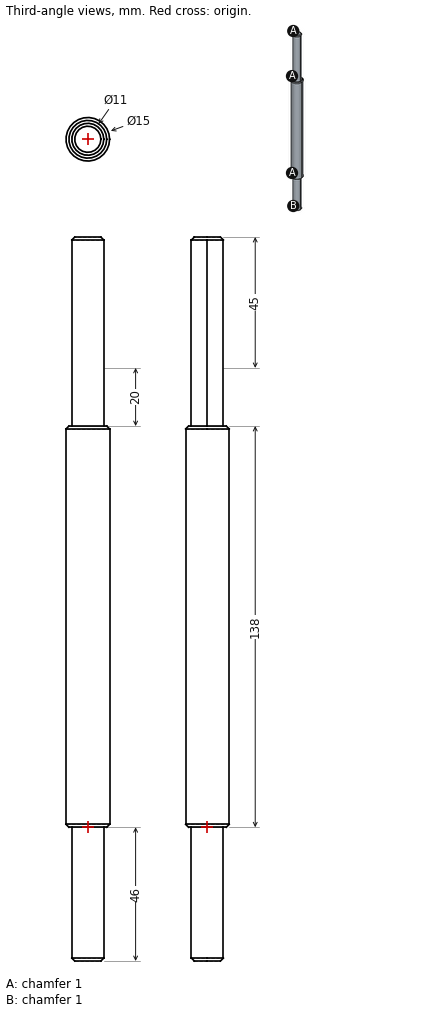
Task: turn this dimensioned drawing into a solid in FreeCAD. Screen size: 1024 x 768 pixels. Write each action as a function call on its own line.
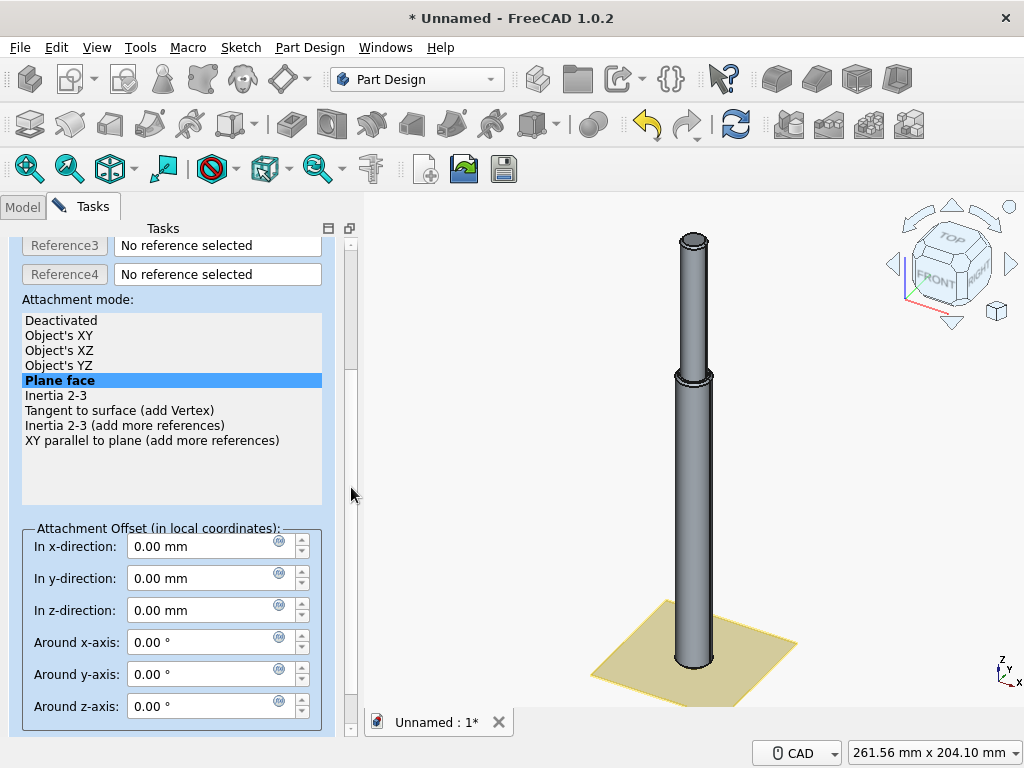
triple_click(210, 610)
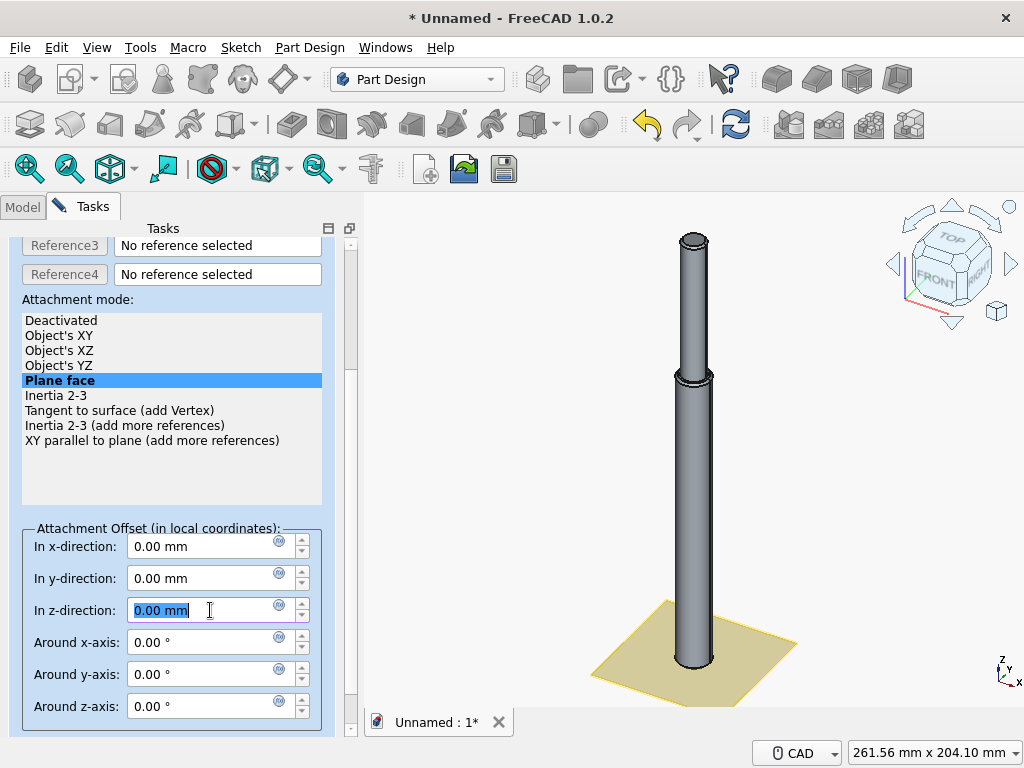
text(-46)
key(Tab)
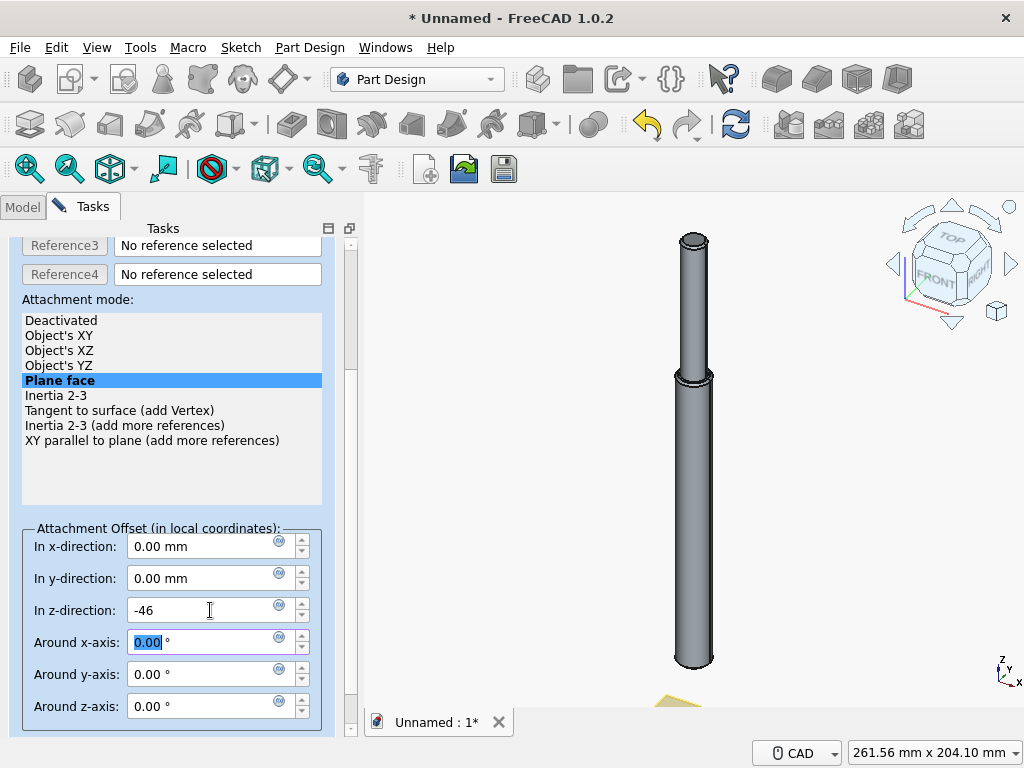
scroll(351, 487, up, 4)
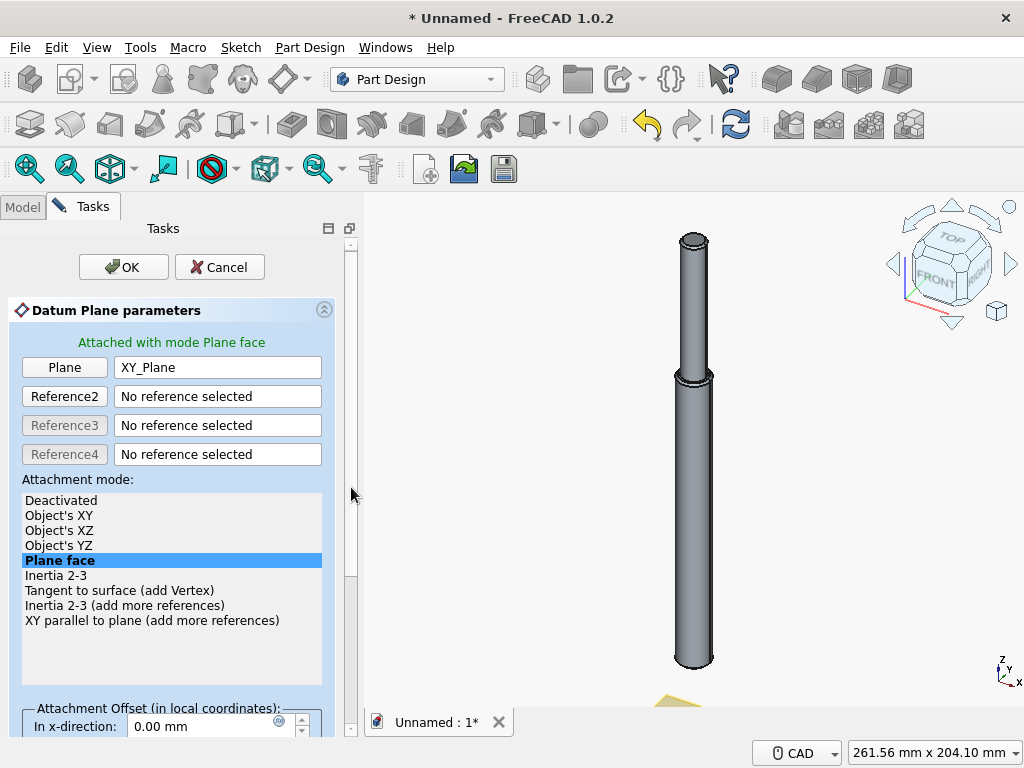
click(124, 267)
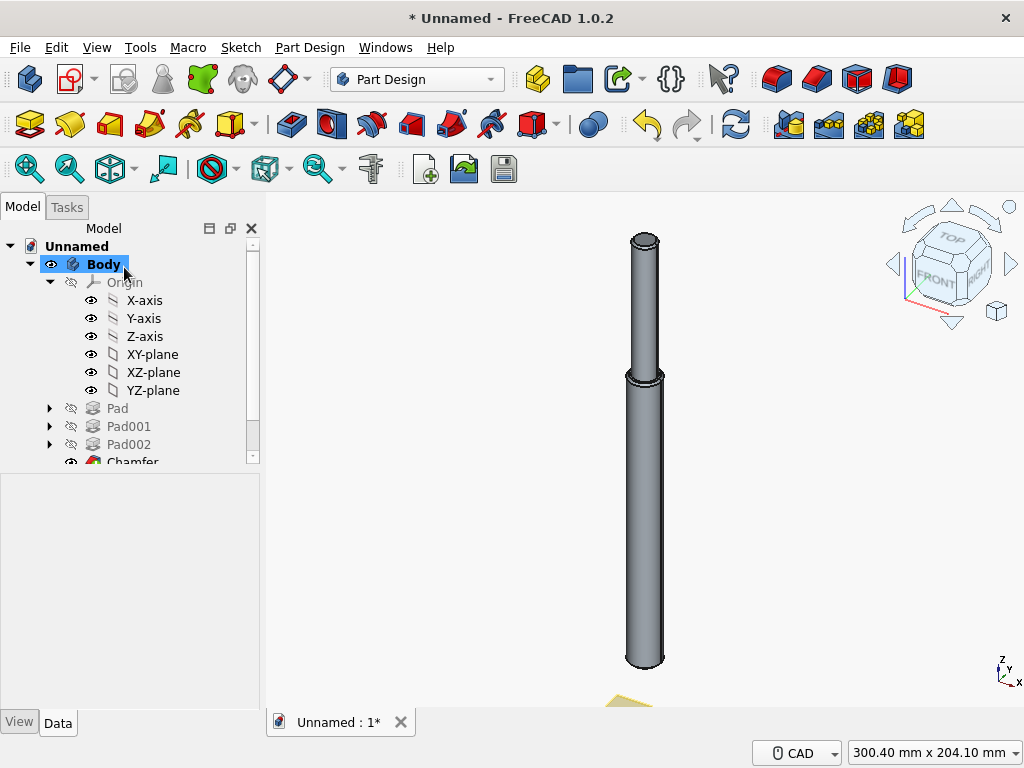
scroll(100, 350, down, 3)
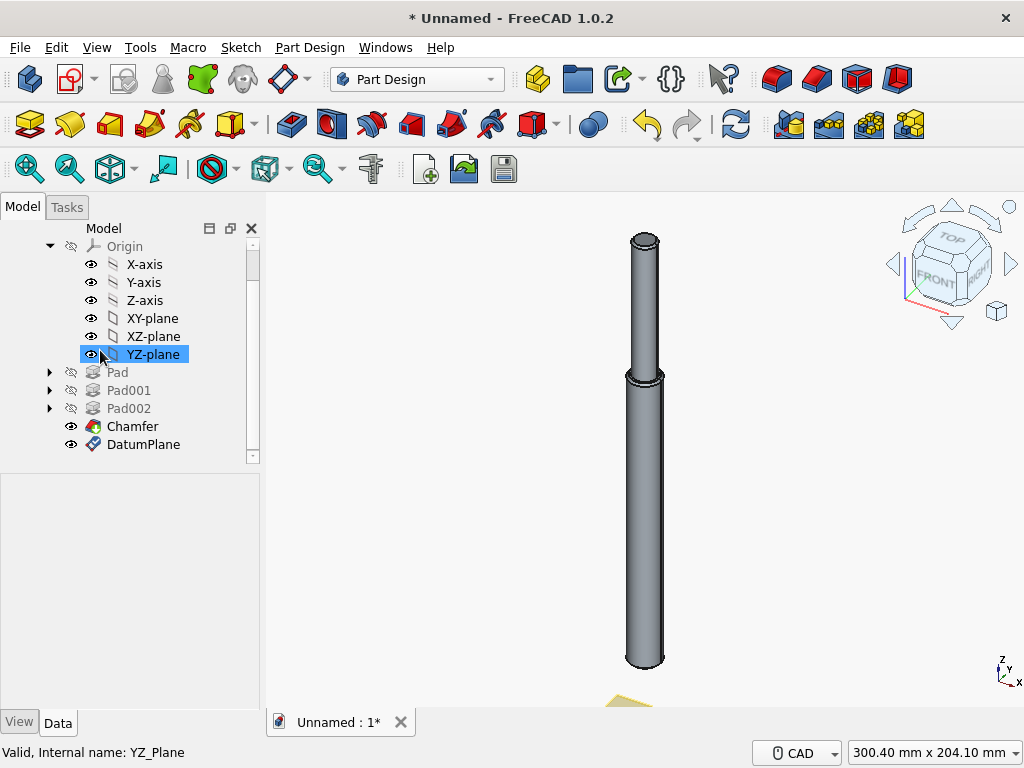
click(116, 444)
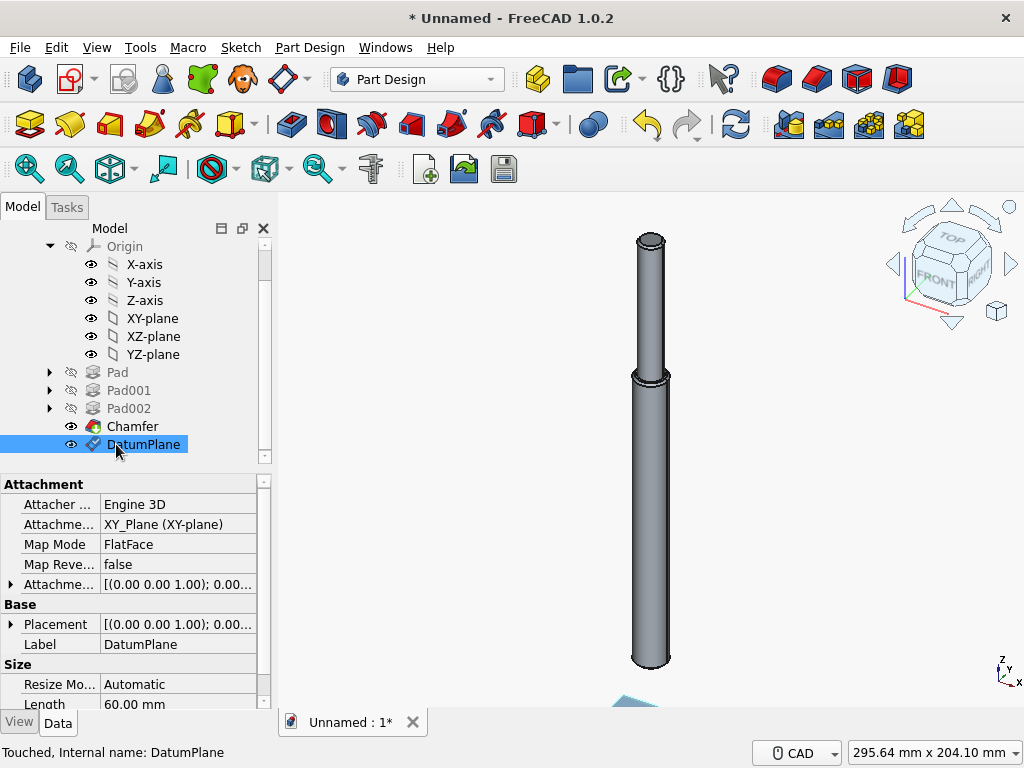
click(70, 80)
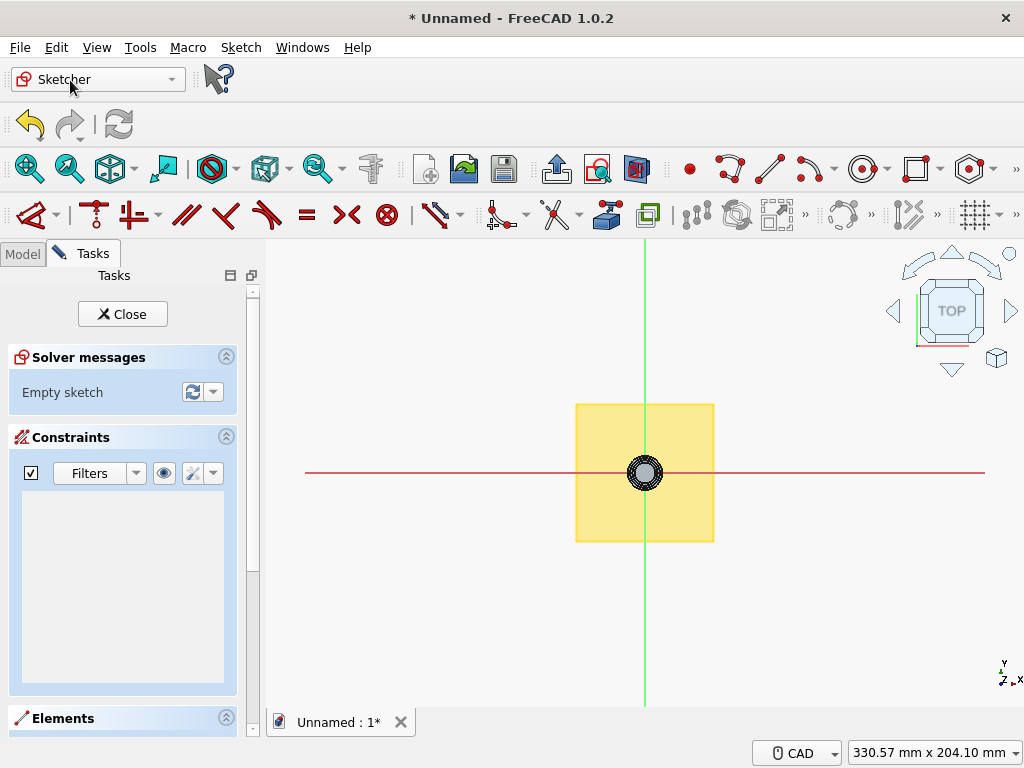
click(638, 170)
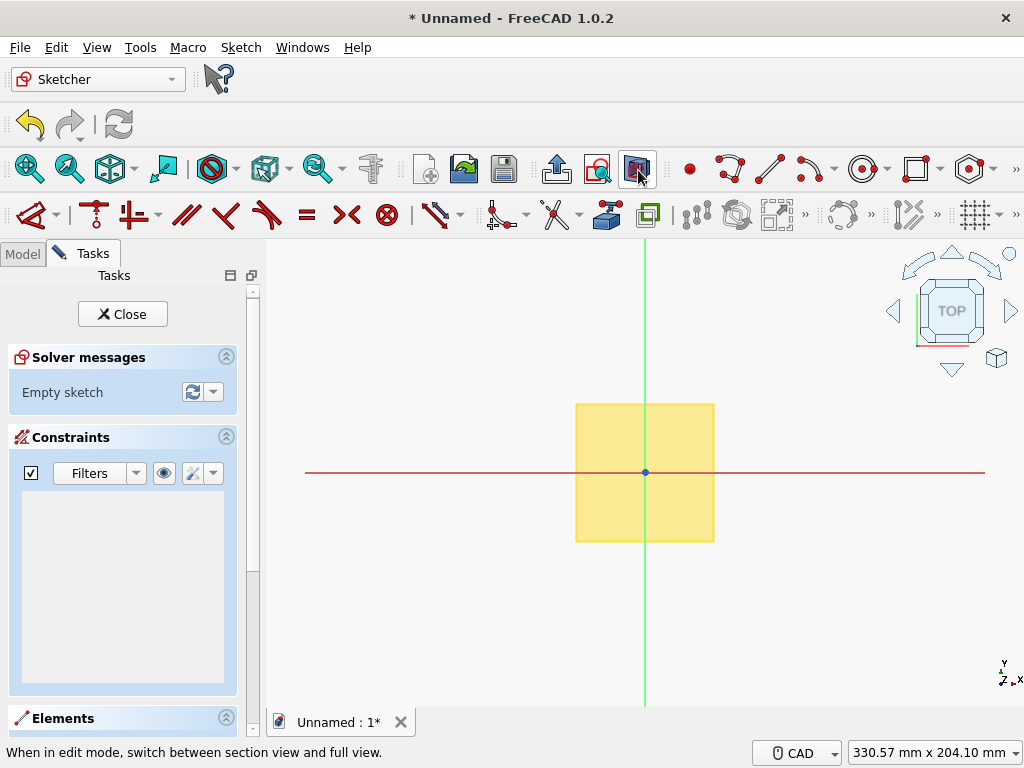
scroll(652, 473, up, 12)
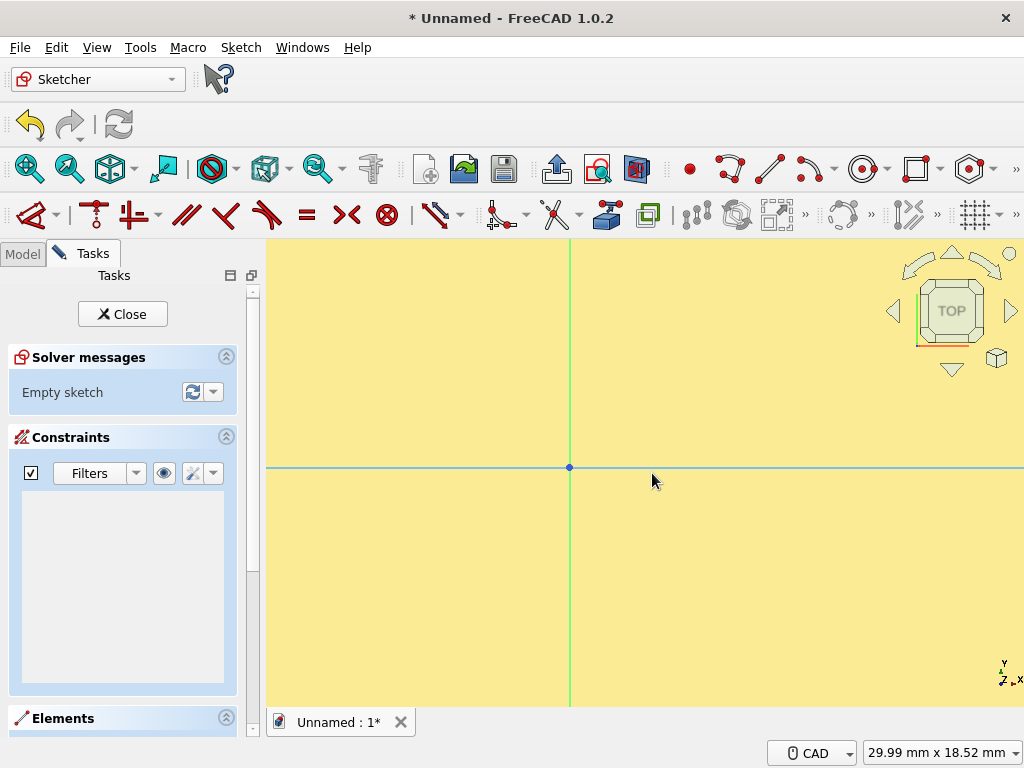
click(864, 170)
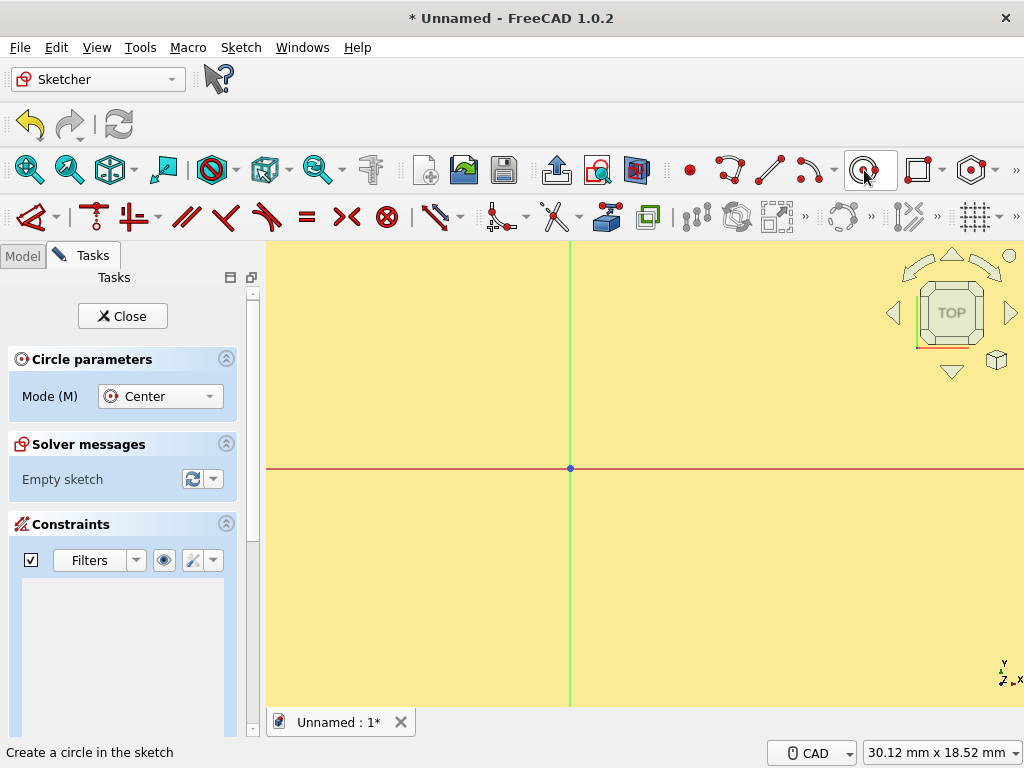
click(570, 469)
click(668, 371)
key(Escape)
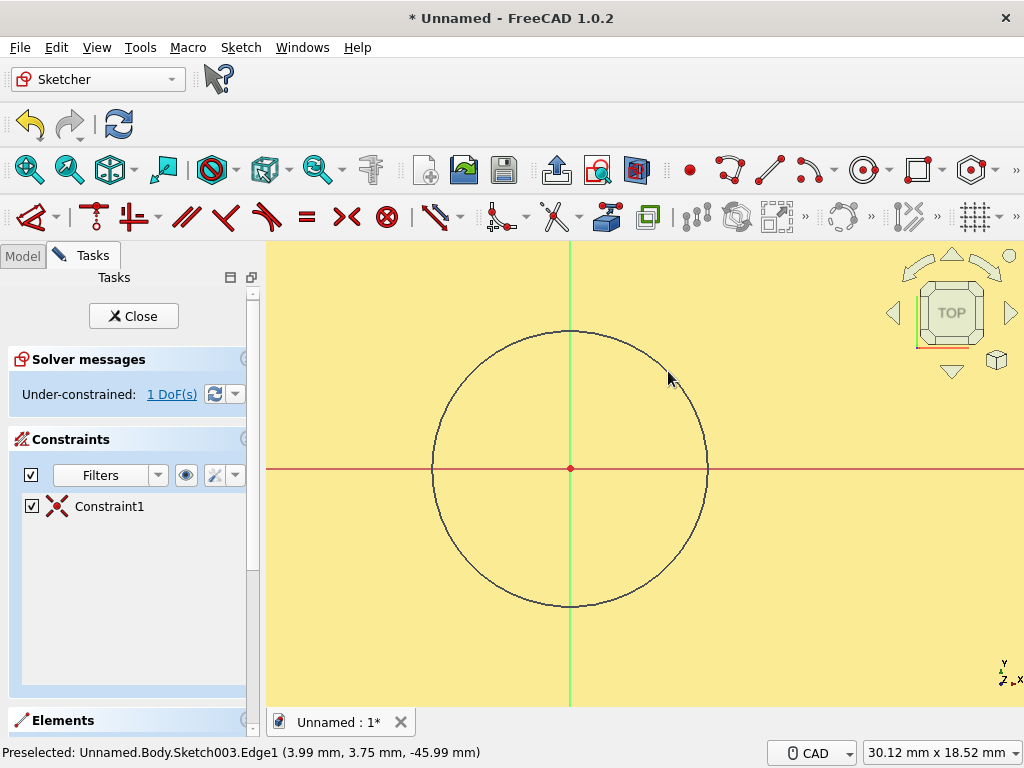
click(32, 218)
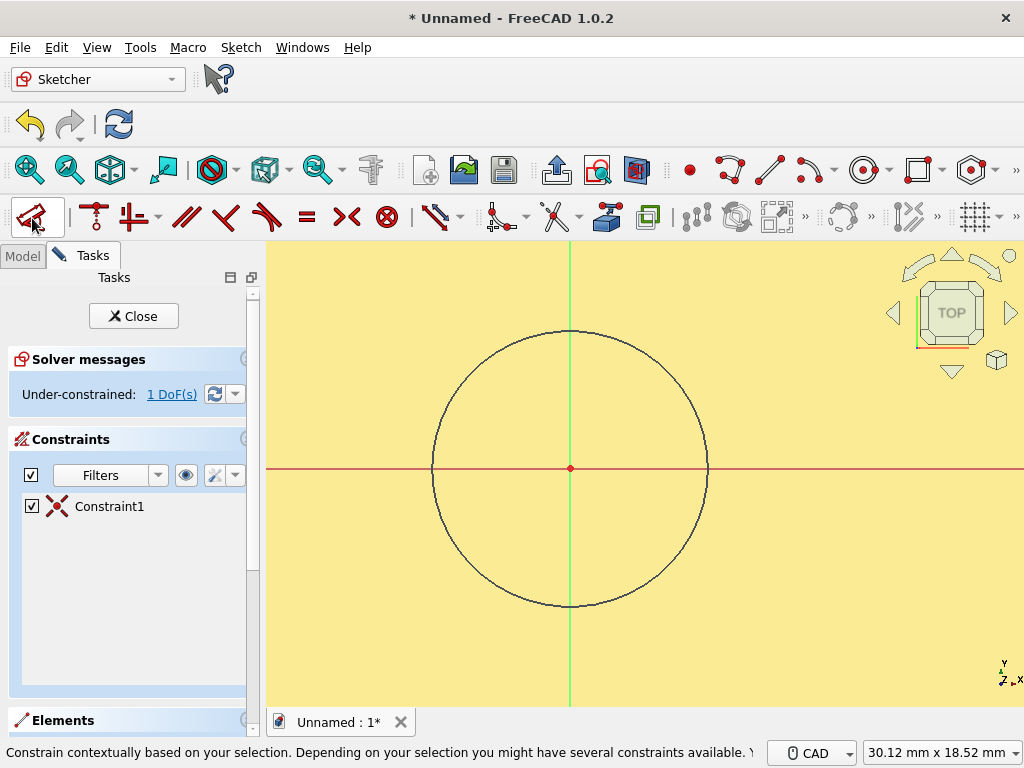
click(667, 371)
click(690, 348)